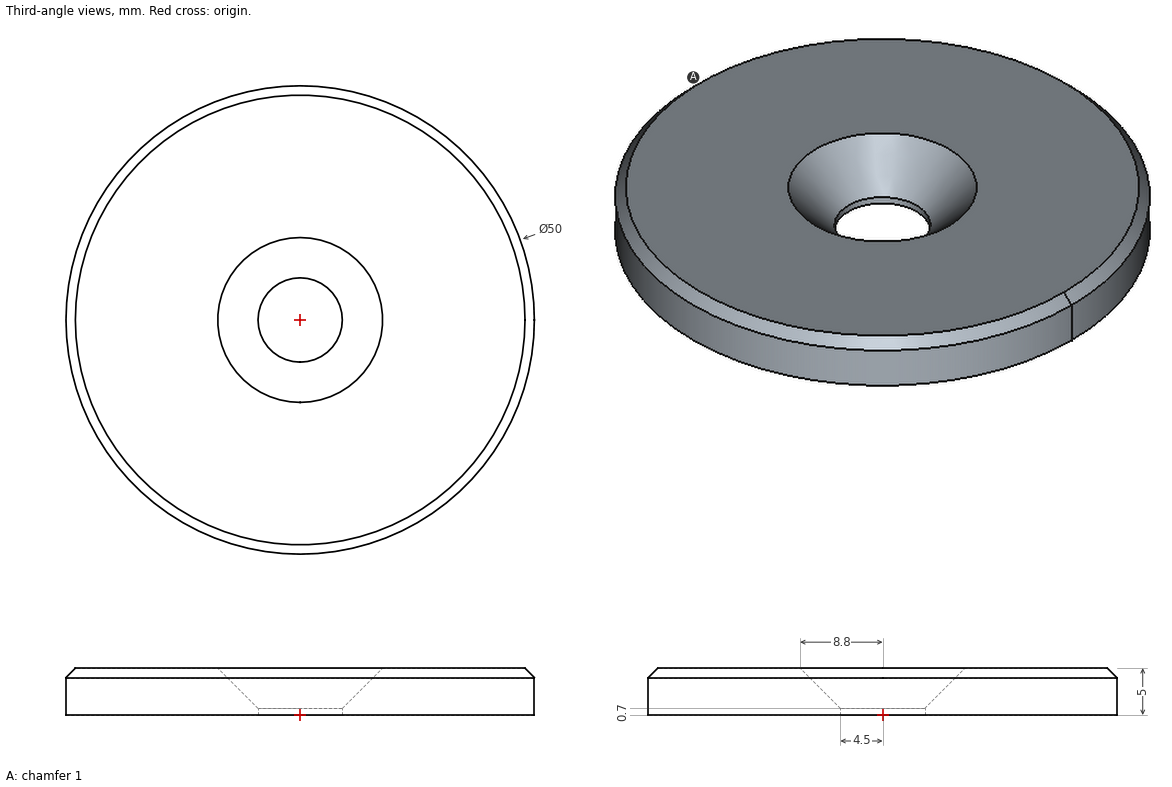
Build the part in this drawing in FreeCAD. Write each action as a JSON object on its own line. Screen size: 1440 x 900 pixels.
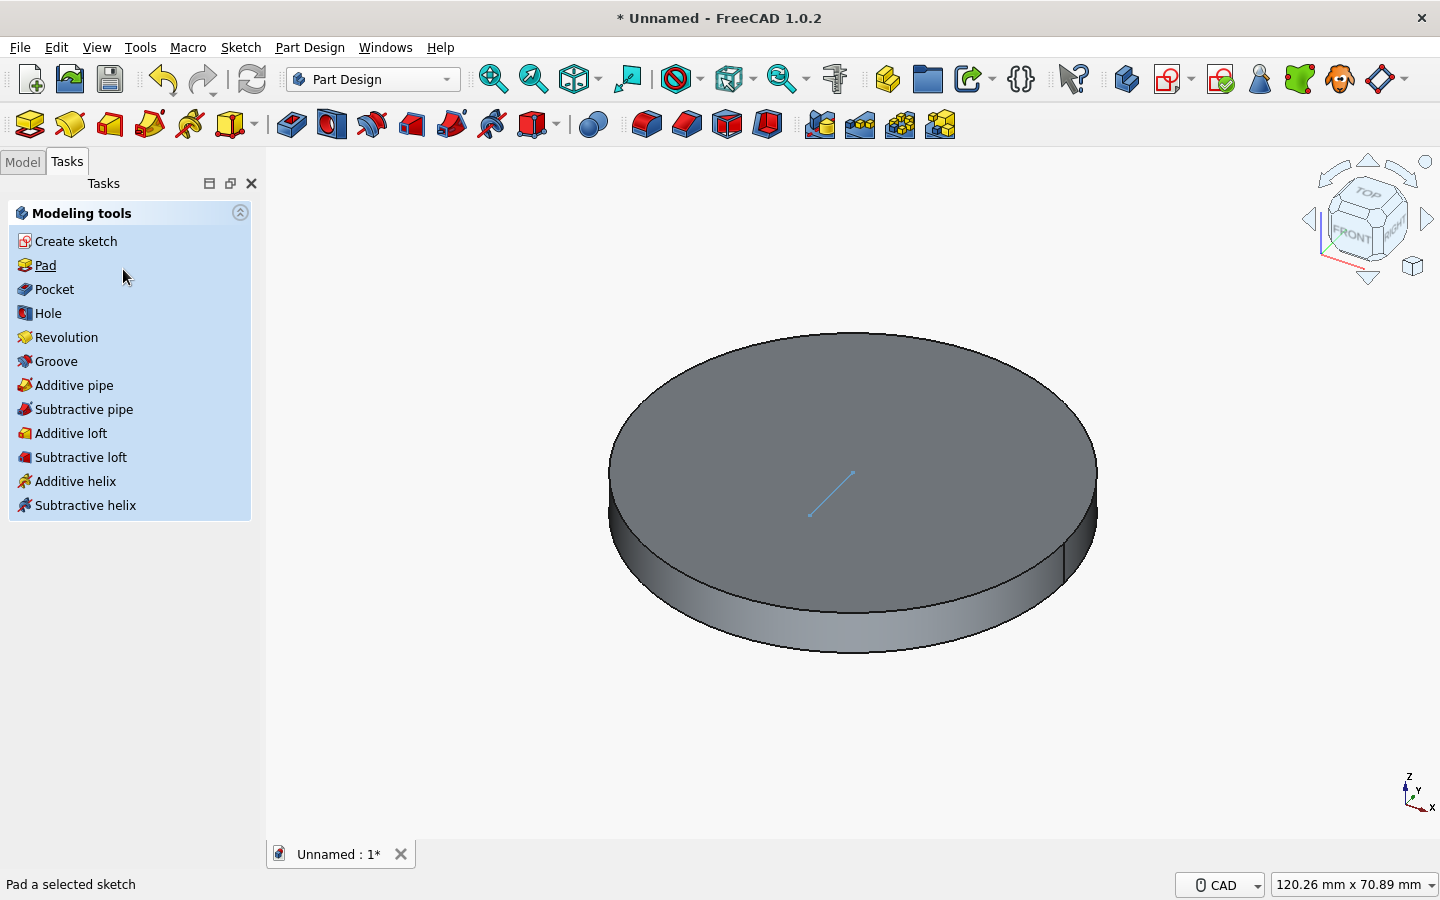
{"action": "left_click", "coordinate": [372, 124]}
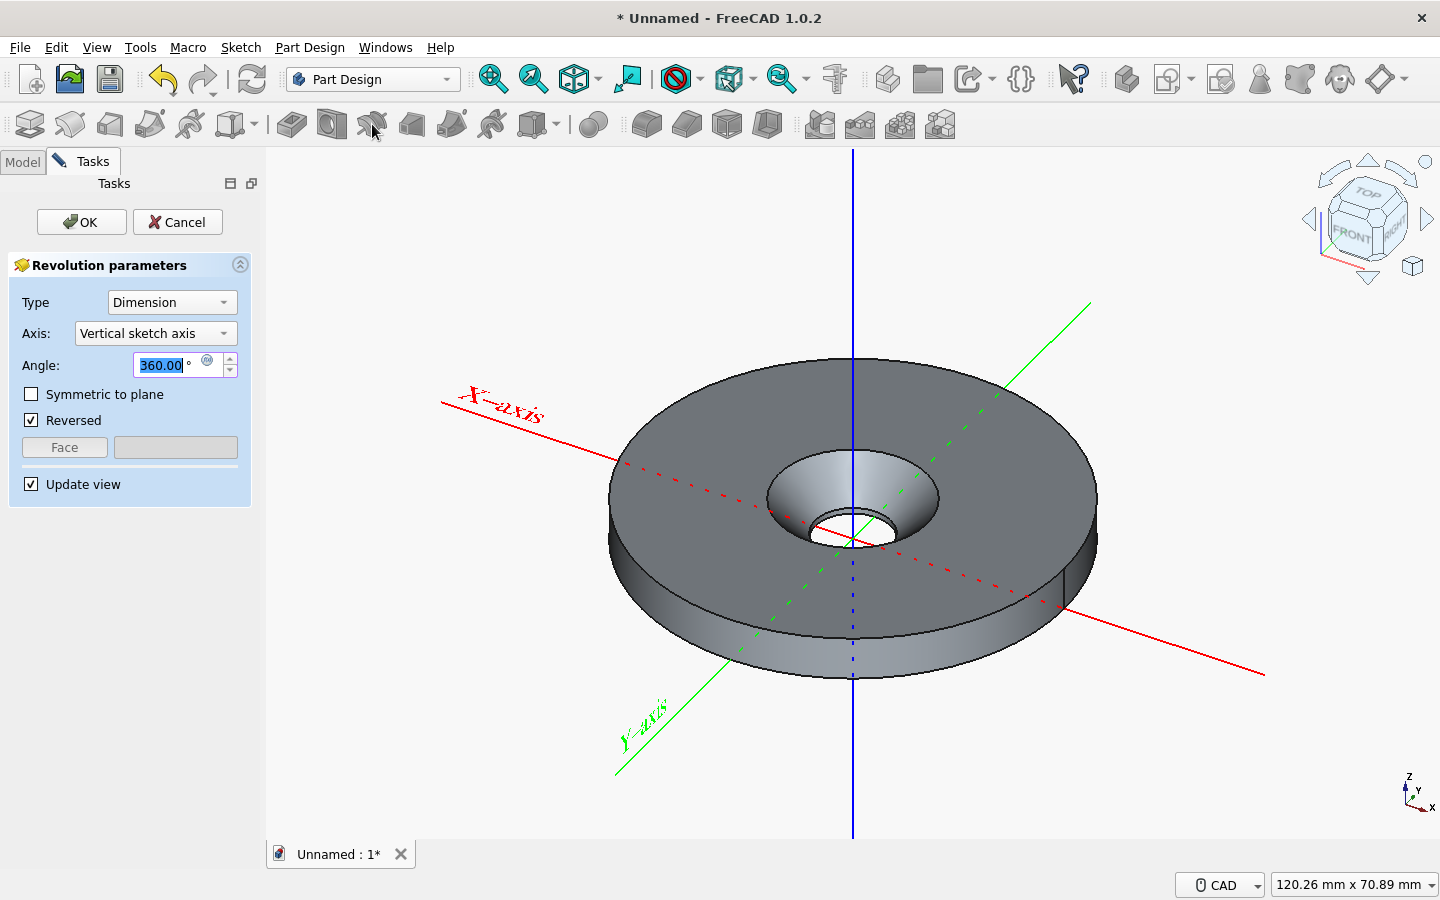
{"action": "left_click", "coordinate": [82, 222]}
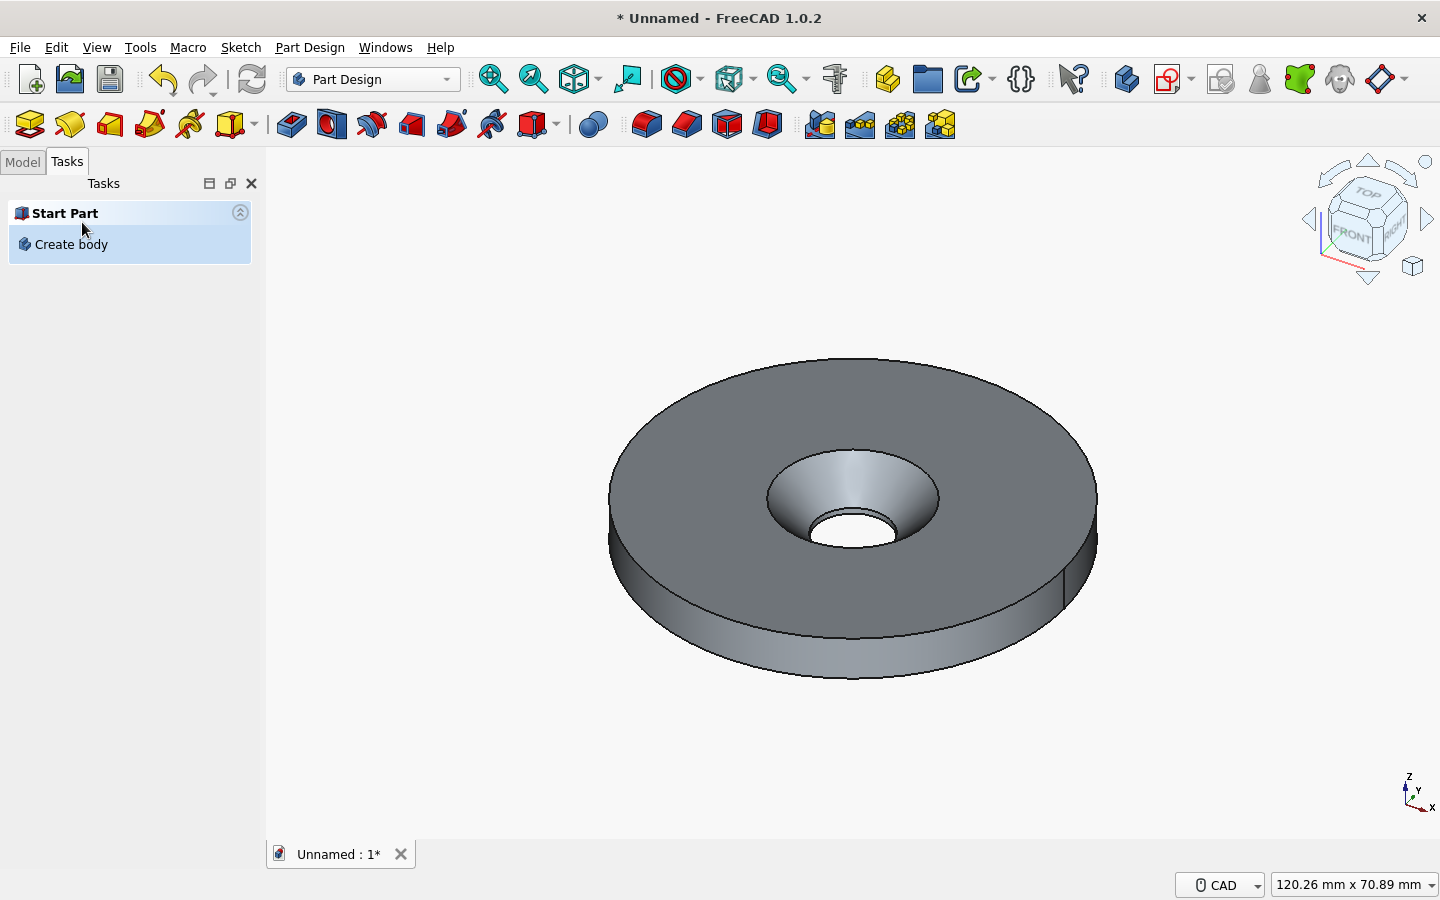
{"action": "left_click", "coordinate": [610, 512]}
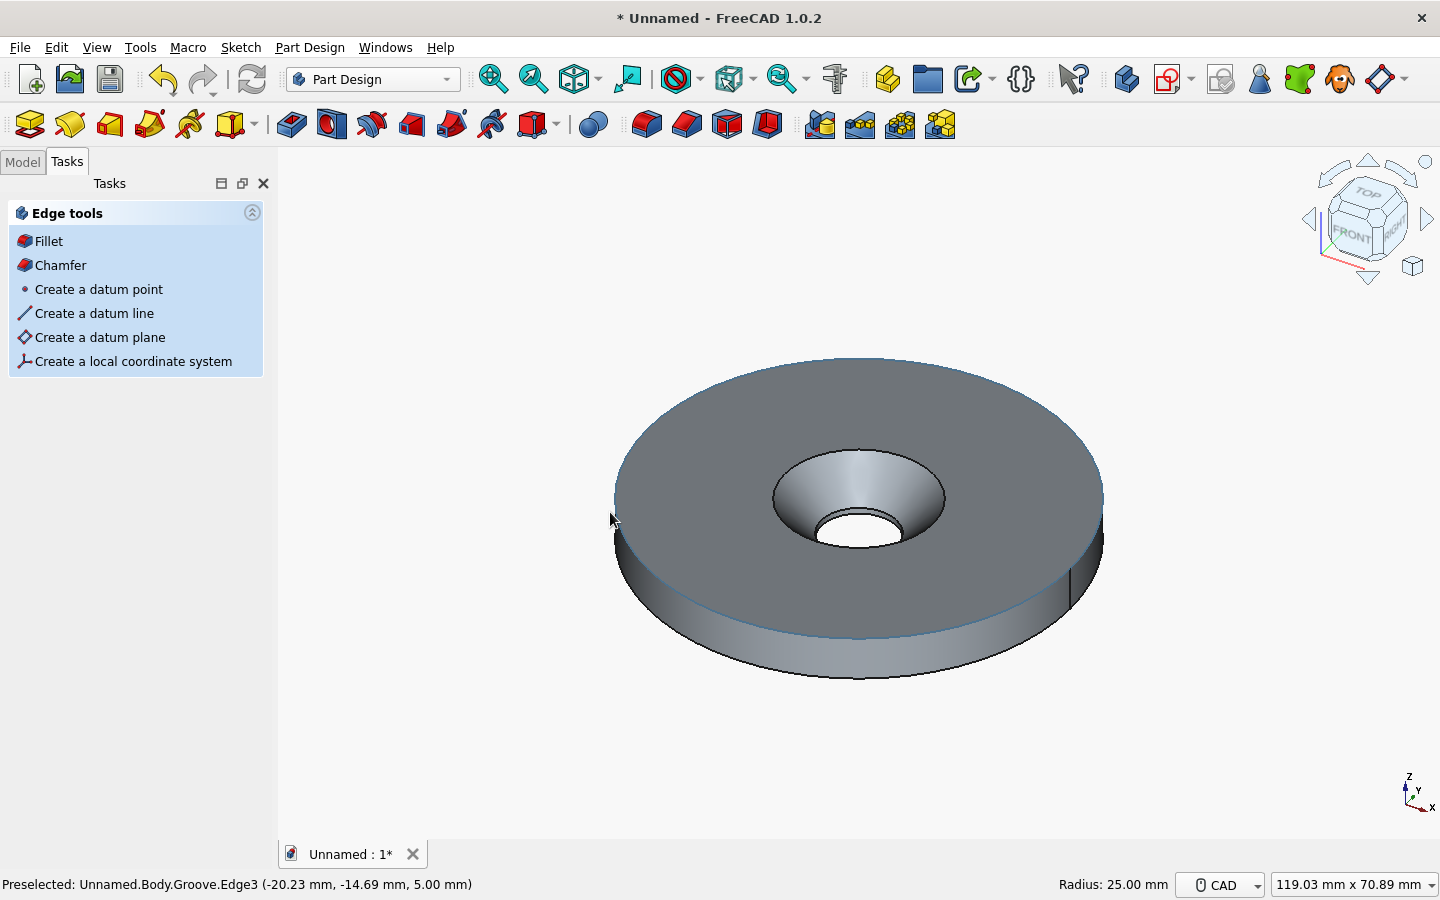
{"action": "left_click", "coordinate": [688, 124]}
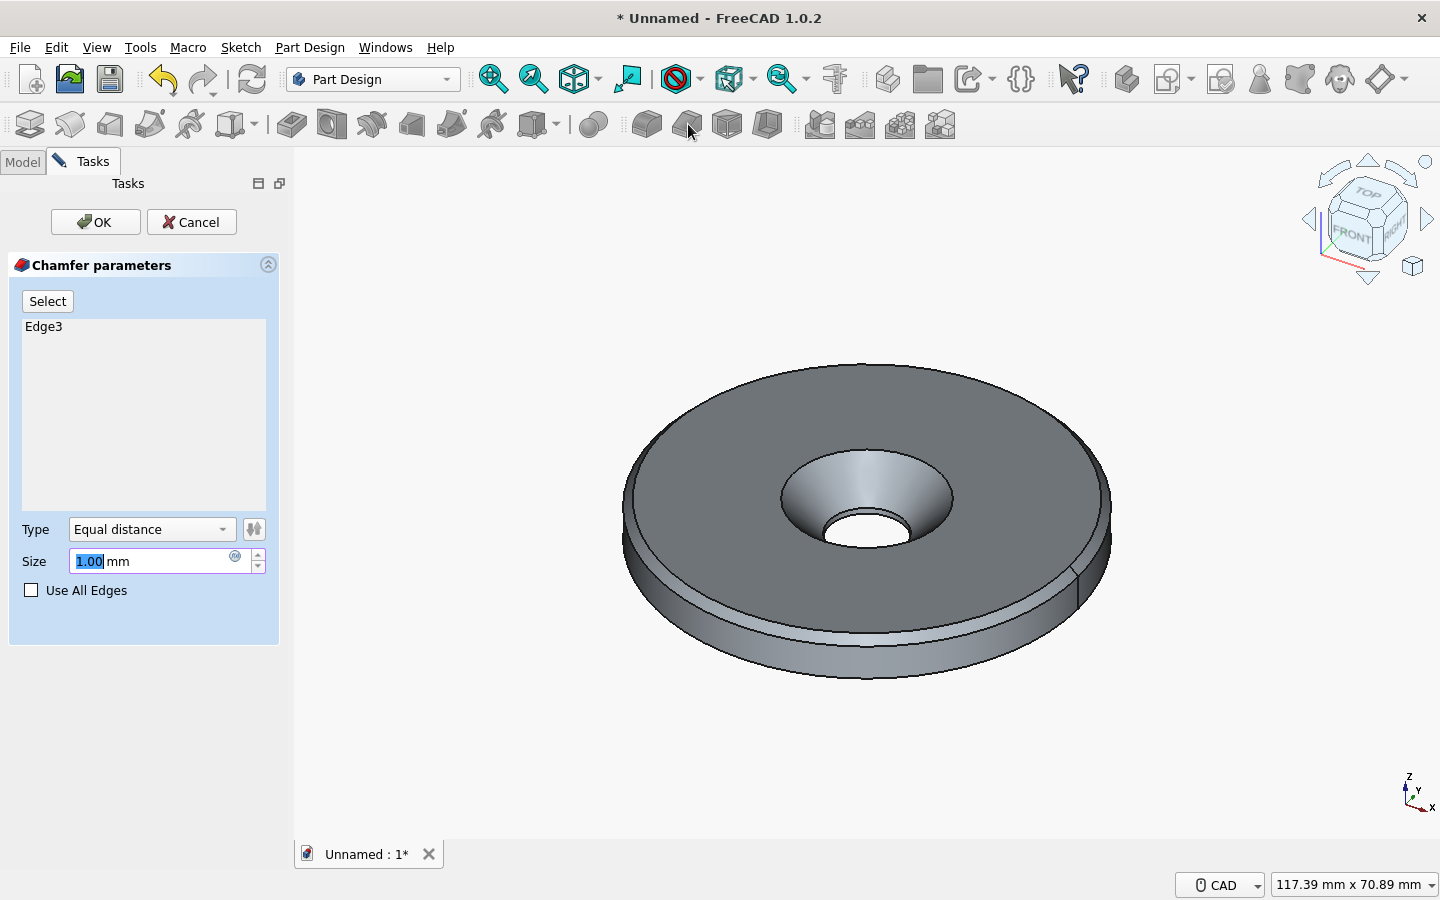
{"action": "type", "text": "1"}
{"action": "key", "text": "Tab"}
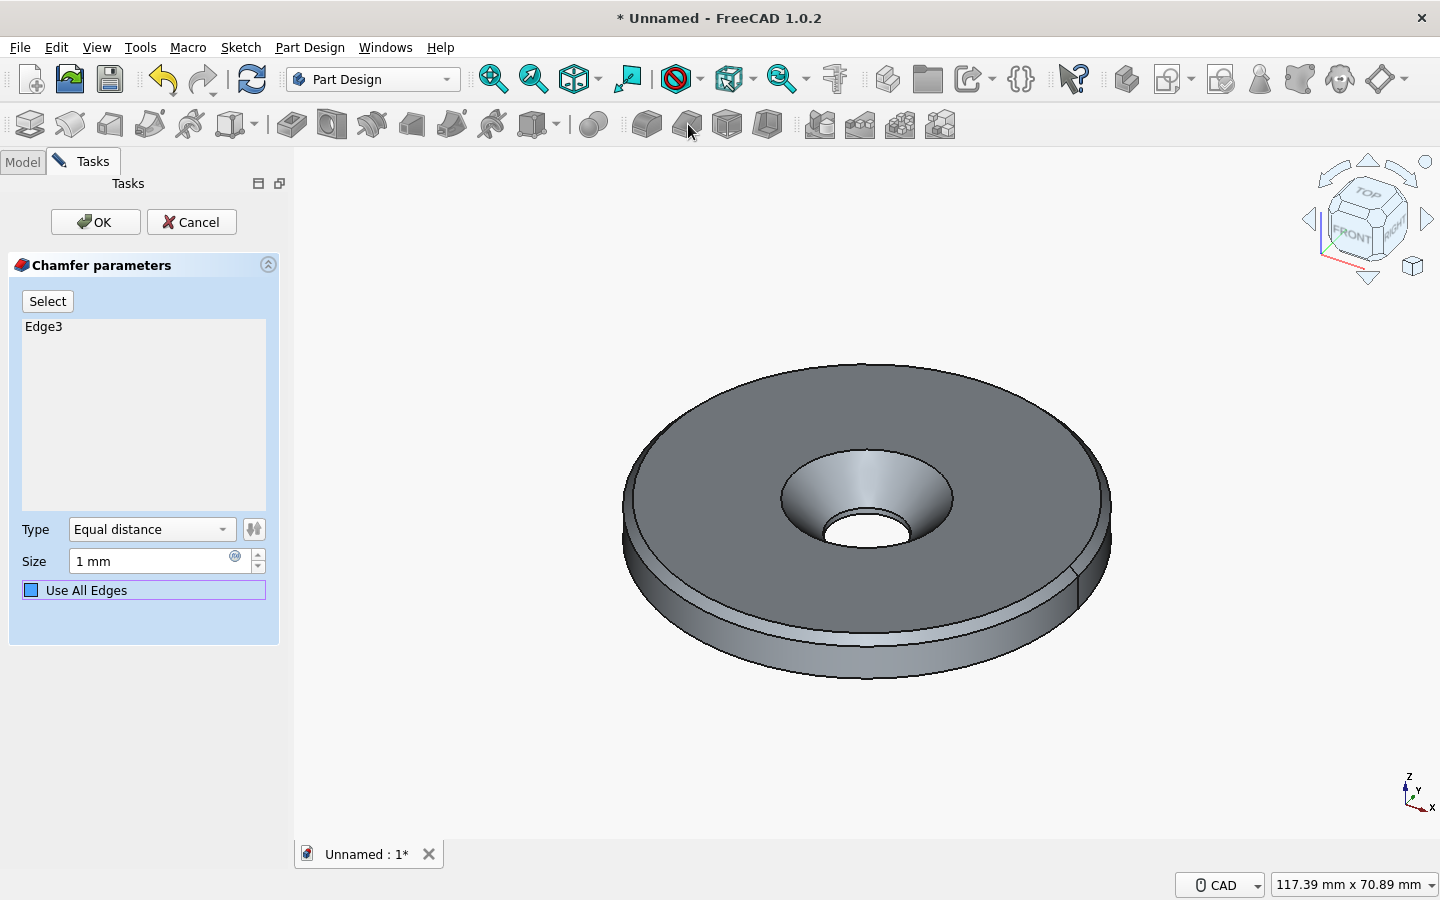
{"action": "left_click", "coordinate": [96, 222]}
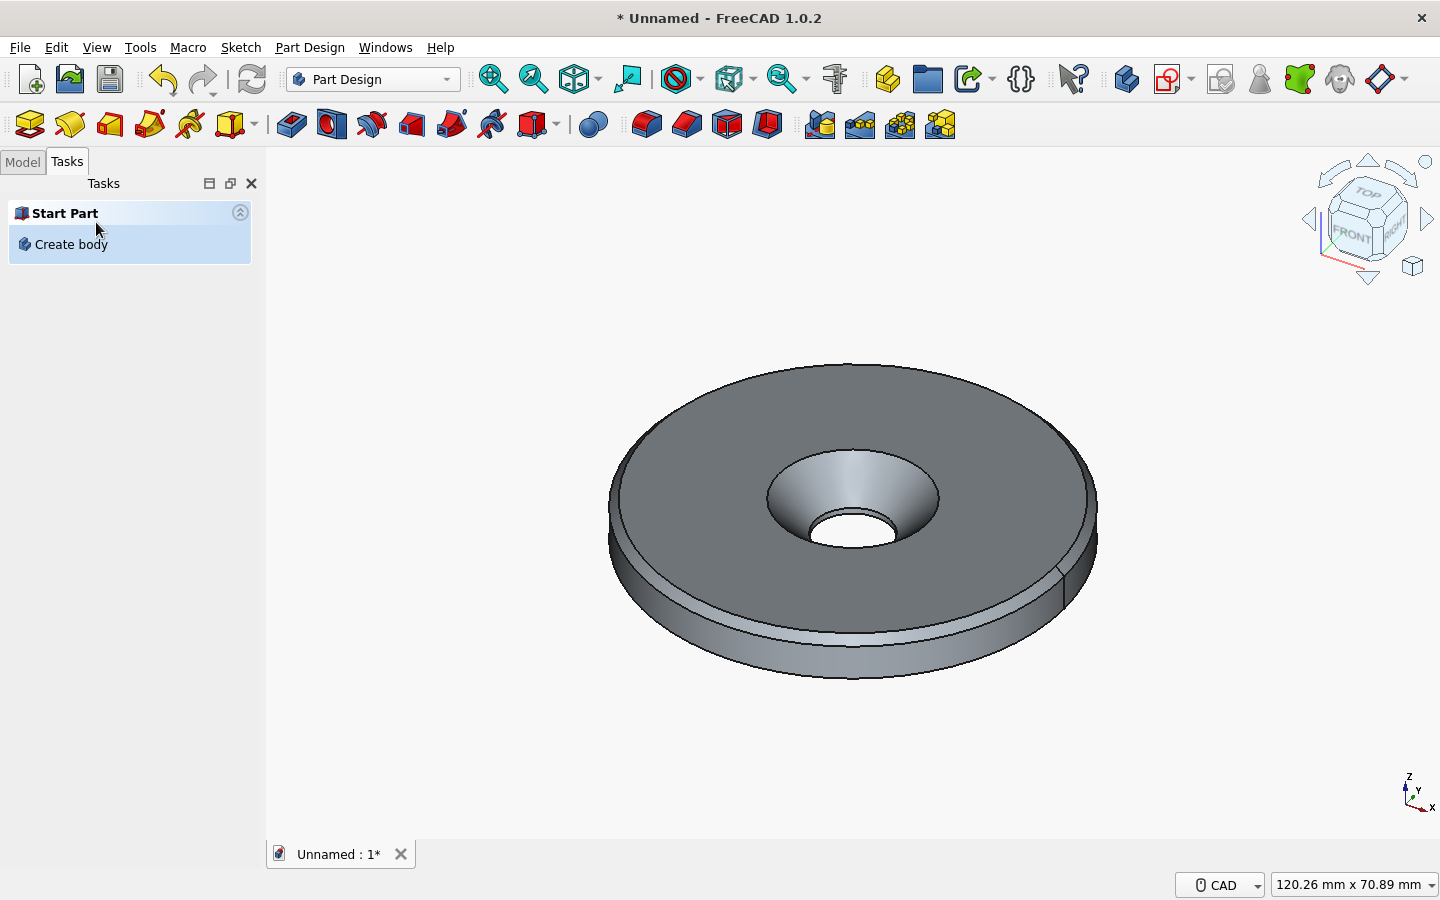
{"action": "key", "text": "0"}